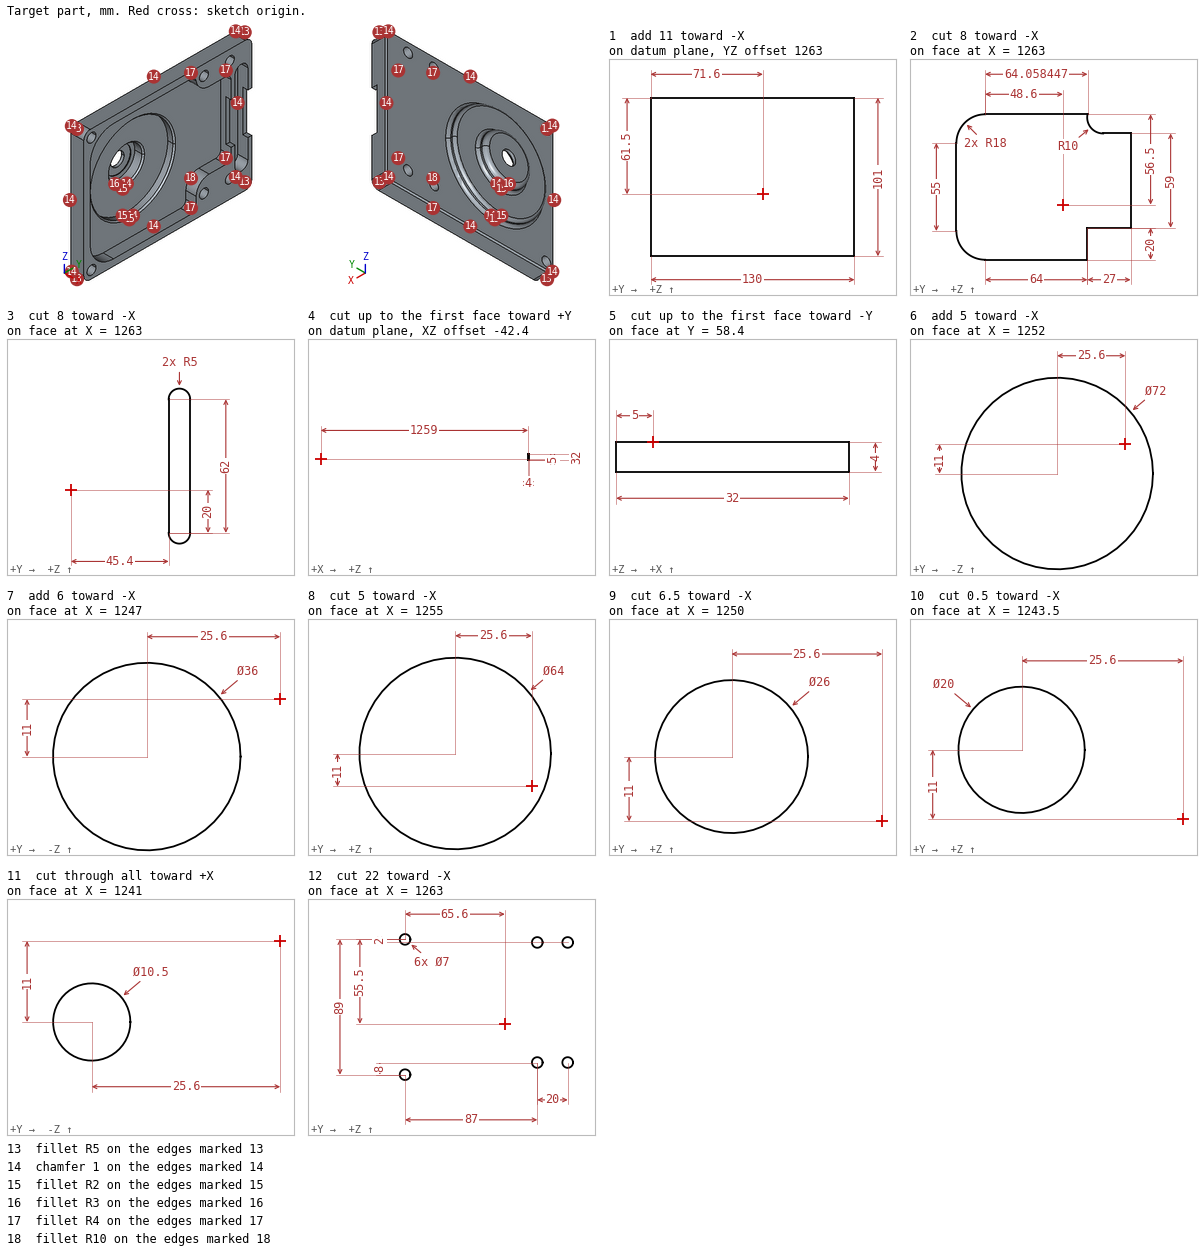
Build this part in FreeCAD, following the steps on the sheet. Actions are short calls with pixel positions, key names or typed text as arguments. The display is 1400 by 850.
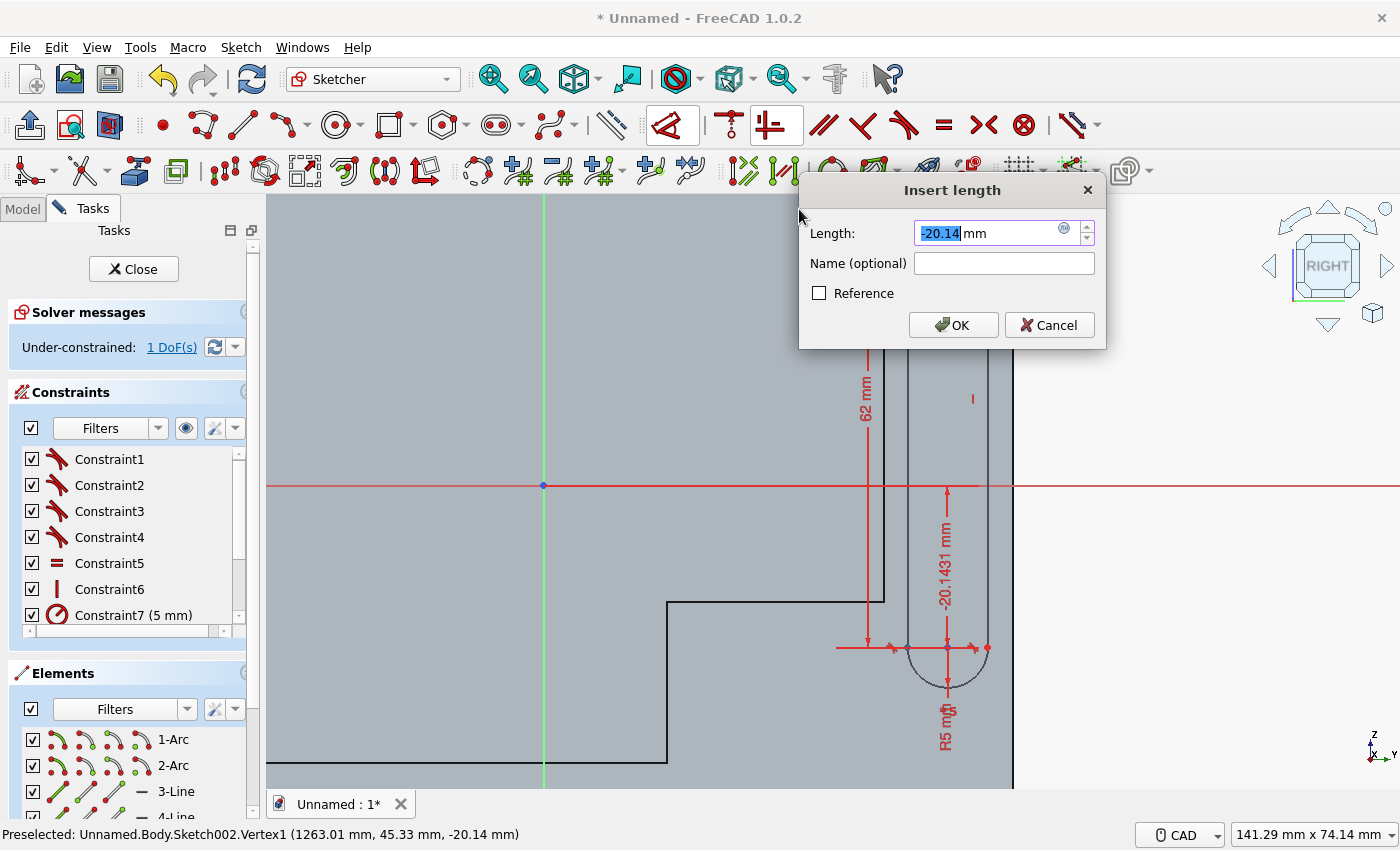
text(-20)
key(Return)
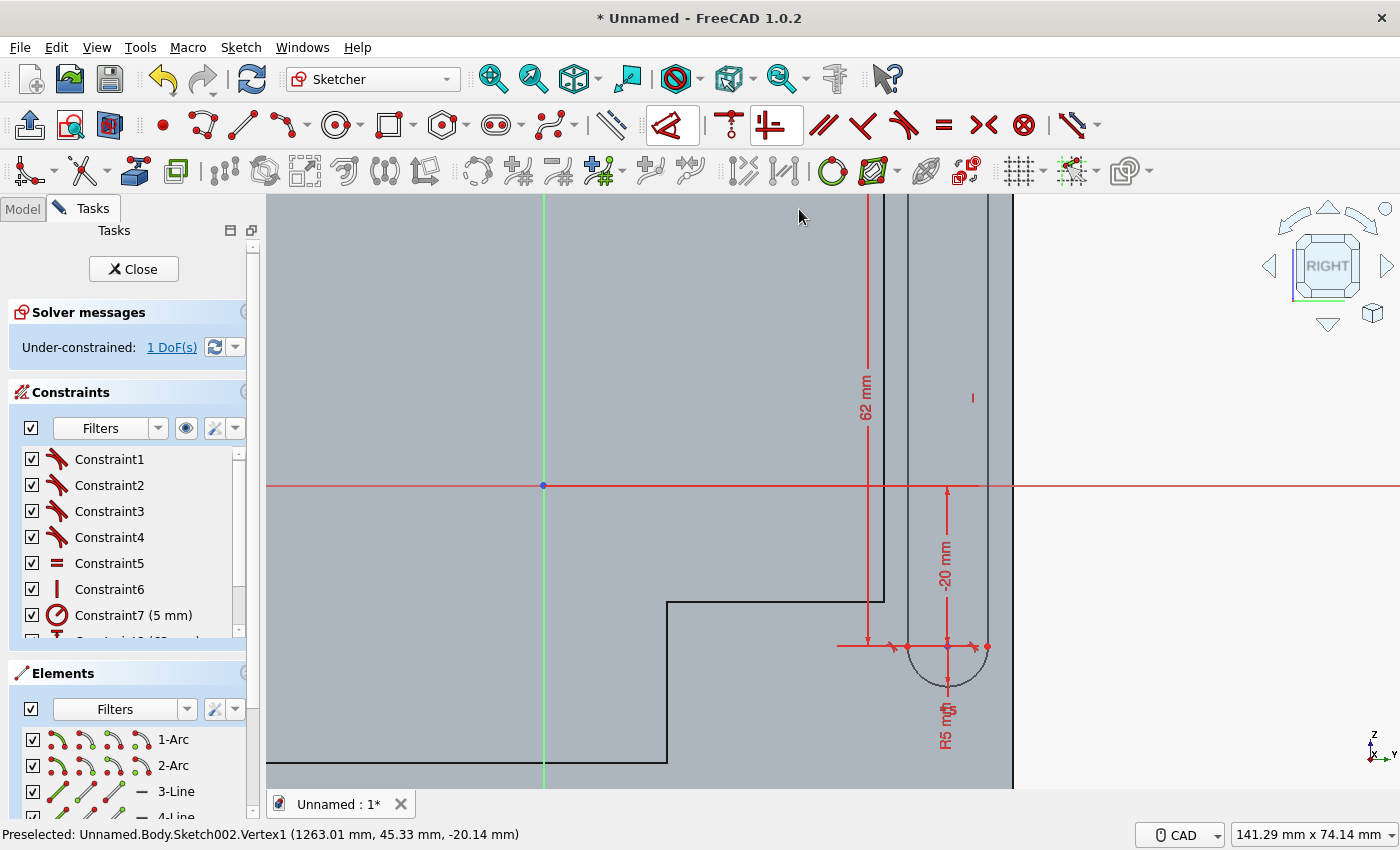
click(908, 646)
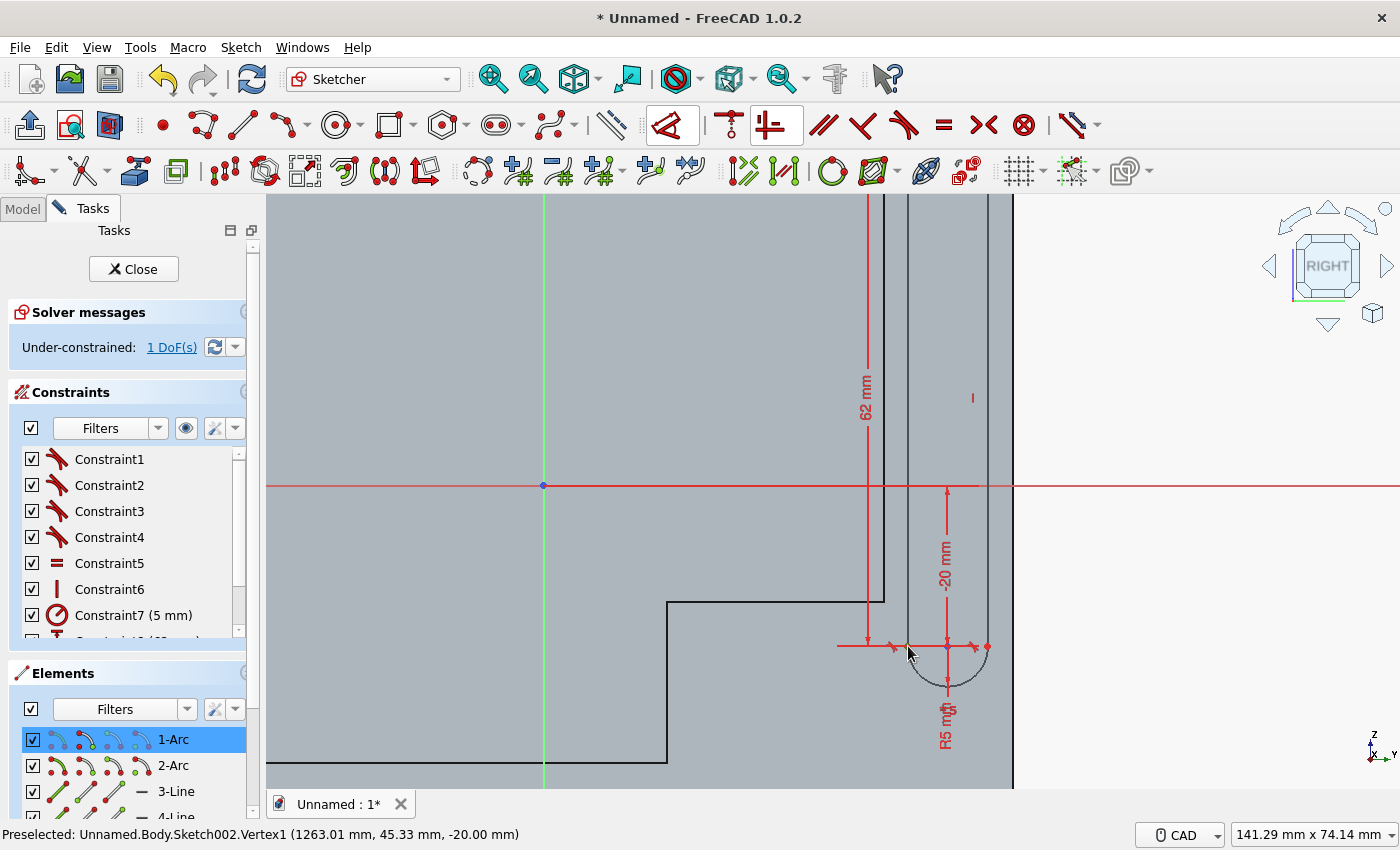
key(l)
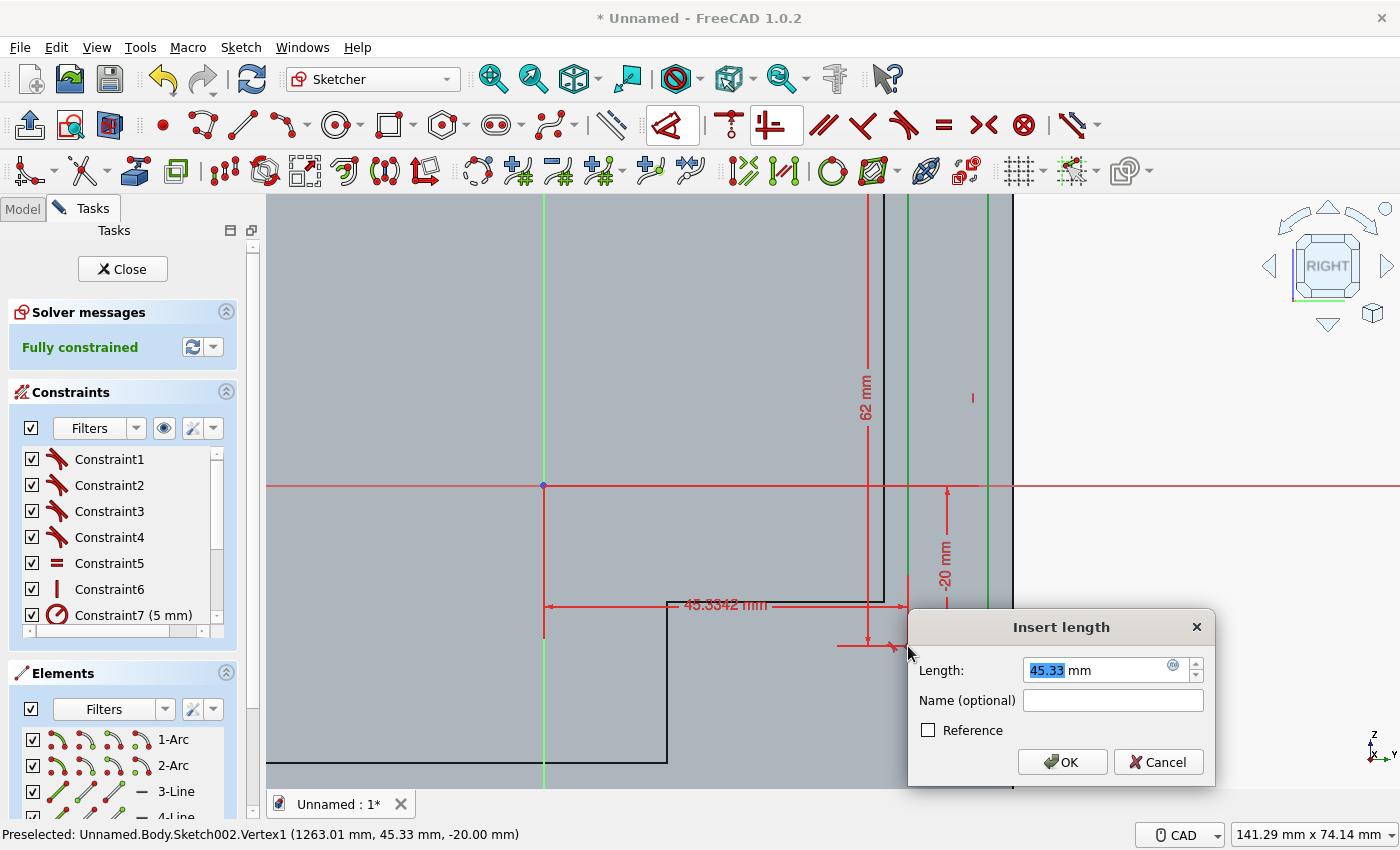
text(45.4)
key(Return)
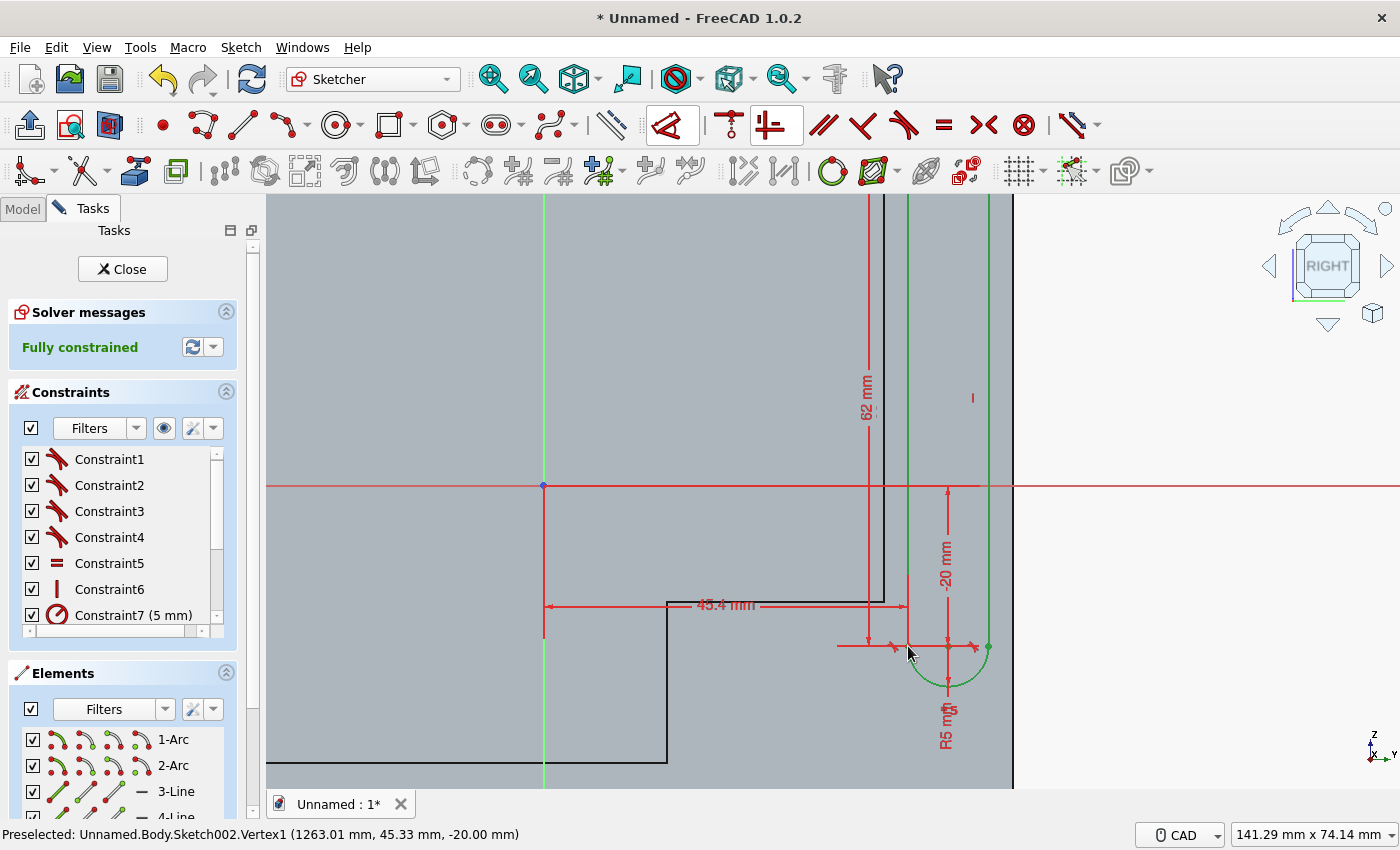
click(123, 269)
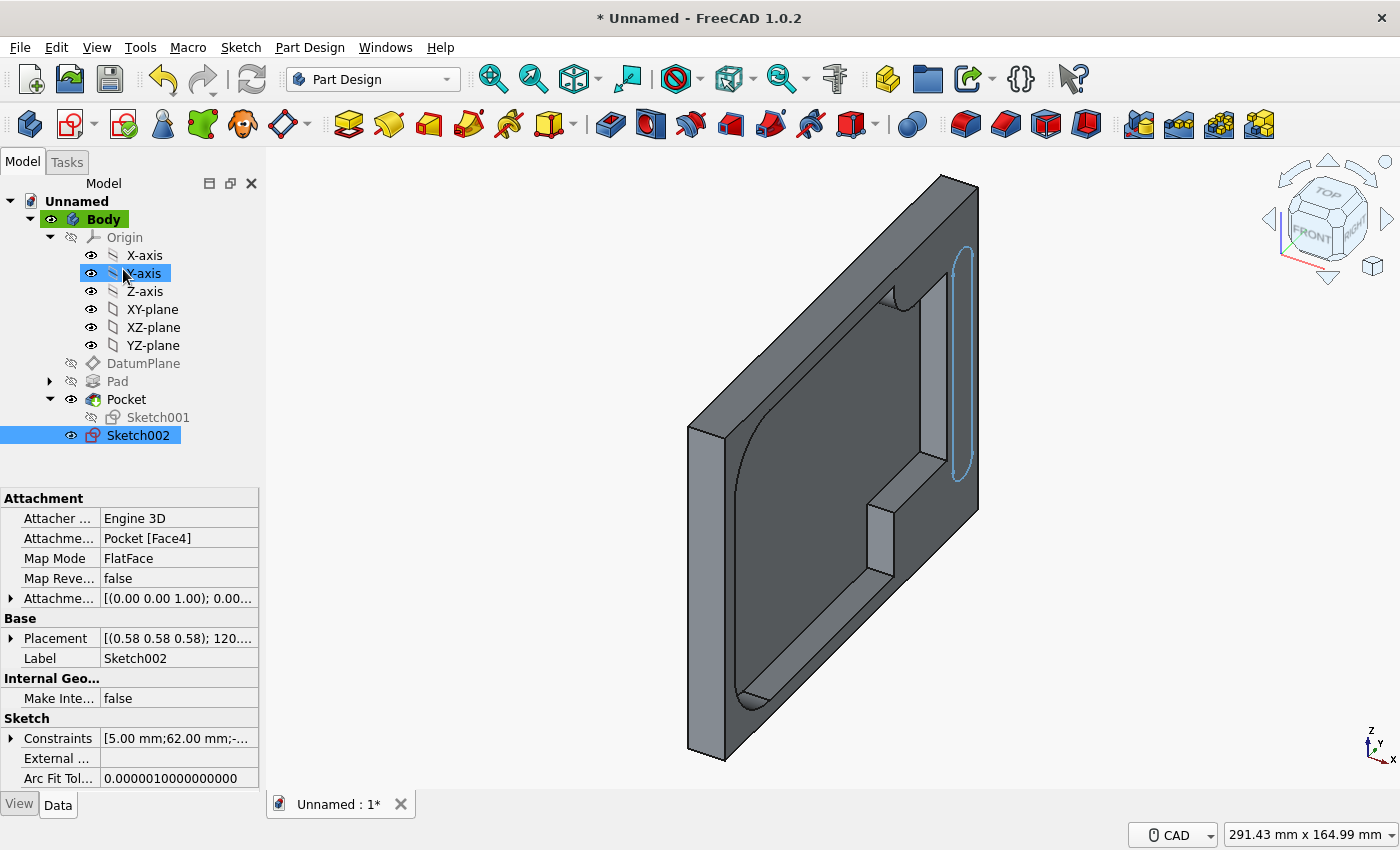
click(612, 124)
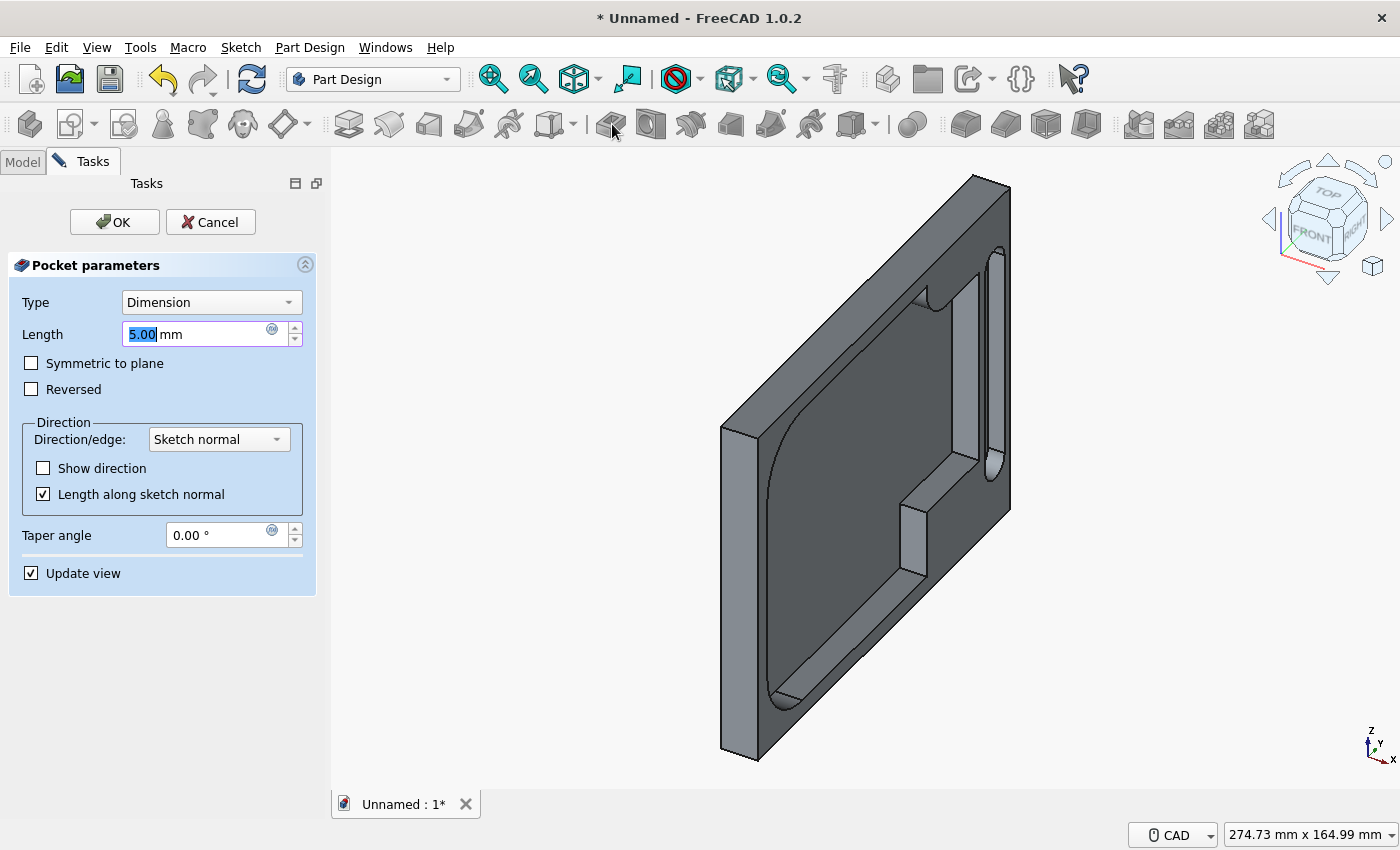
text(8)
key(Tab)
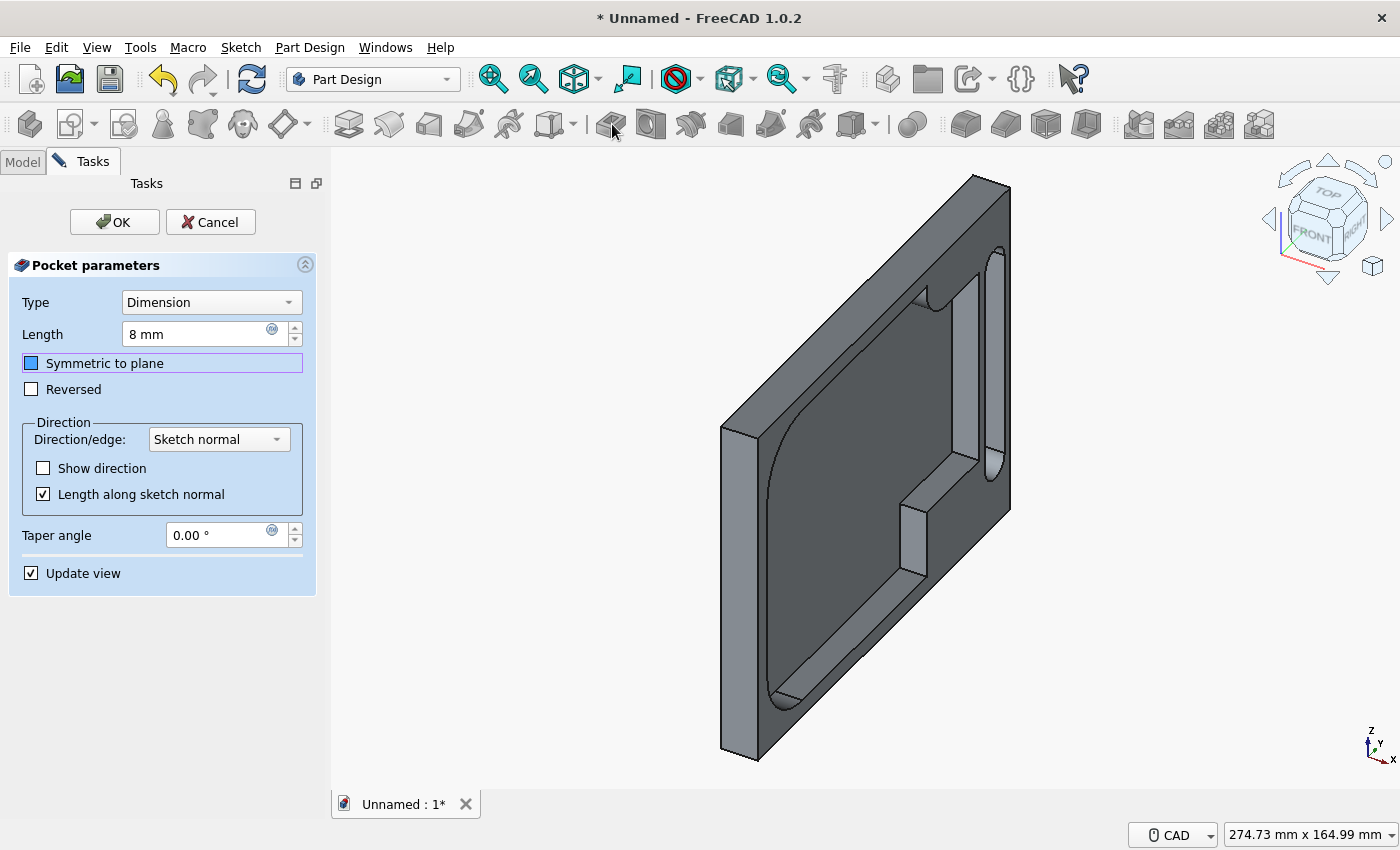
click(115, 222)